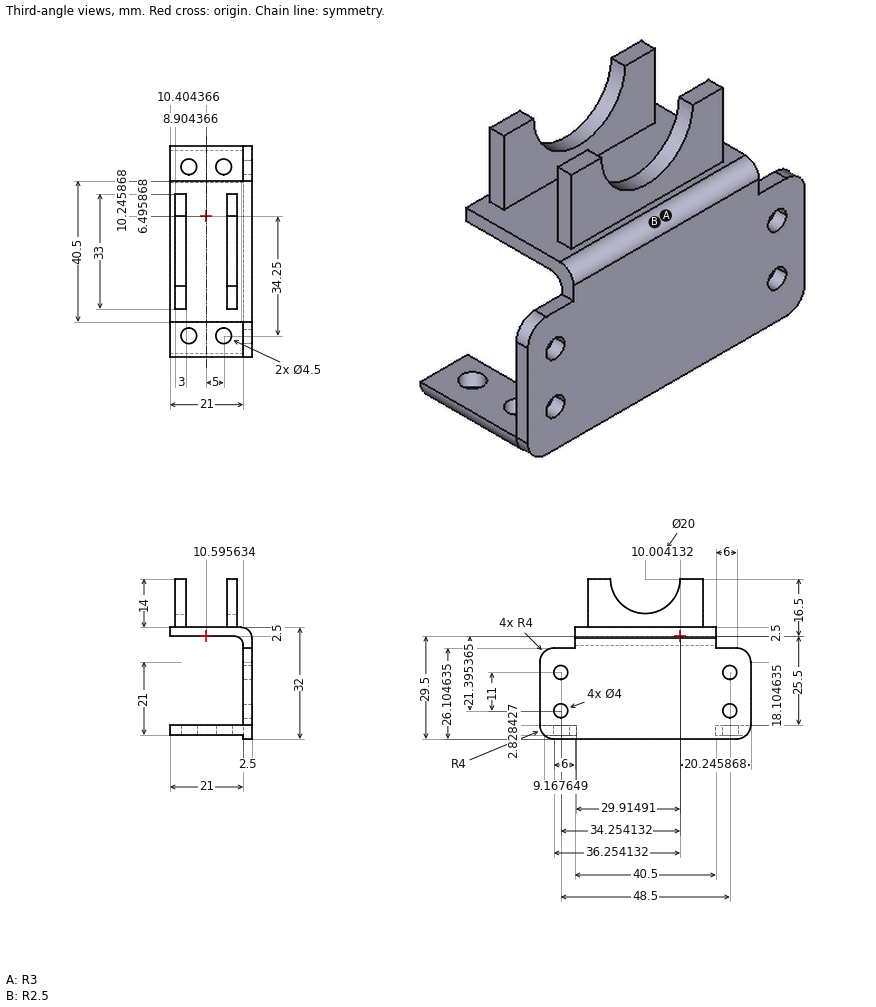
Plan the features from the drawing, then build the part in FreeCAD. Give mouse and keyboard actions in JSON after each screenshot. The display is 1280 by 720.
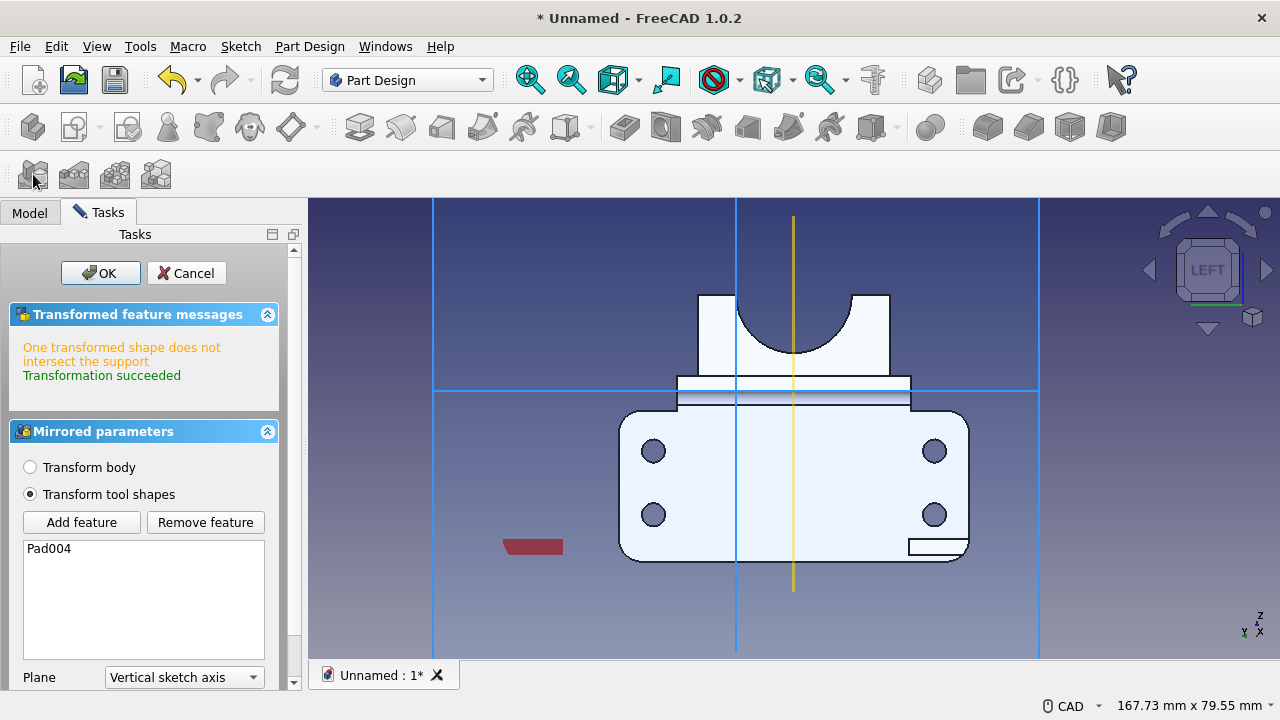
{"action": "left_click", "coordinate": [185, 678]}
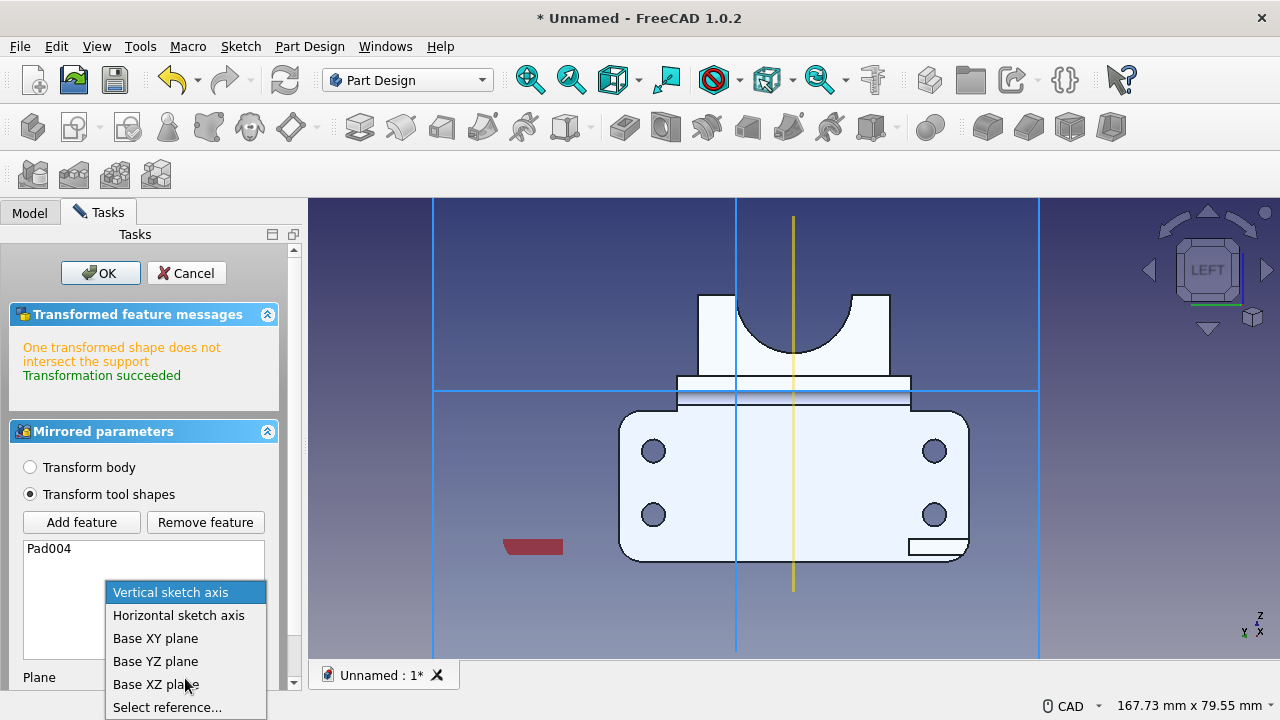
{"action": "left_click", "coordinate": [184, 708]}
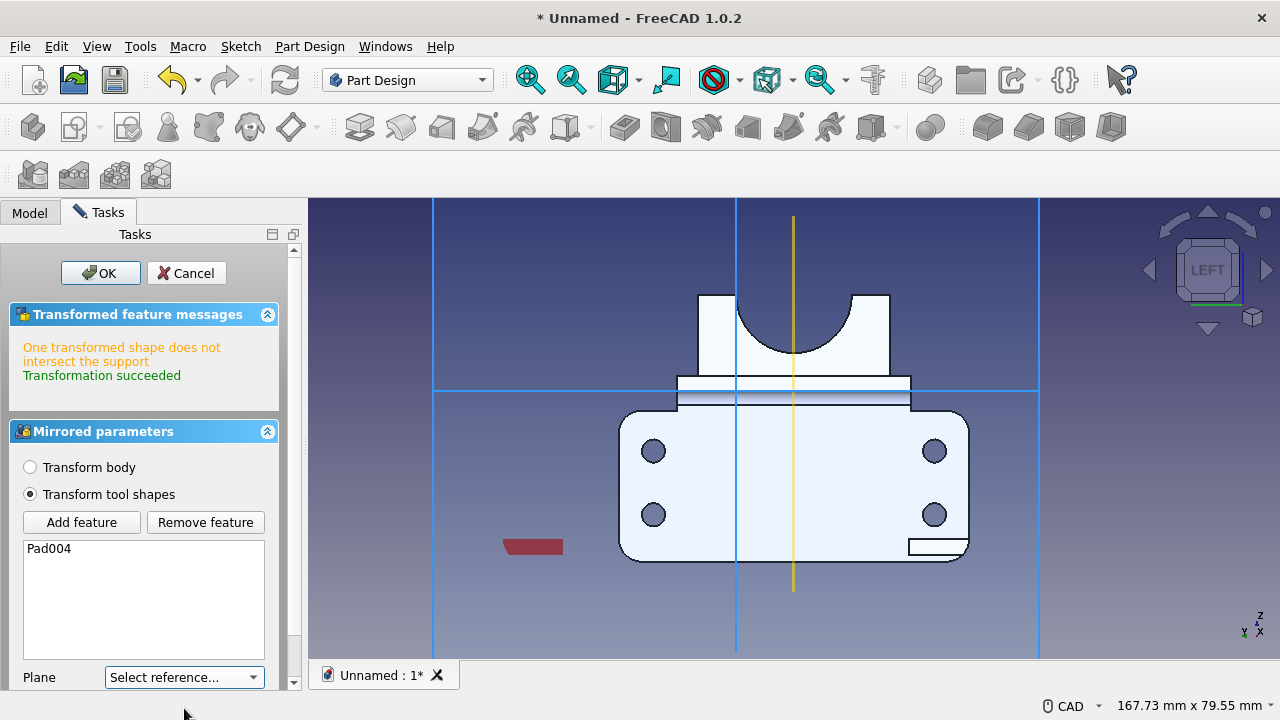
{"action": "left_click", "coordinate": [30, 212]}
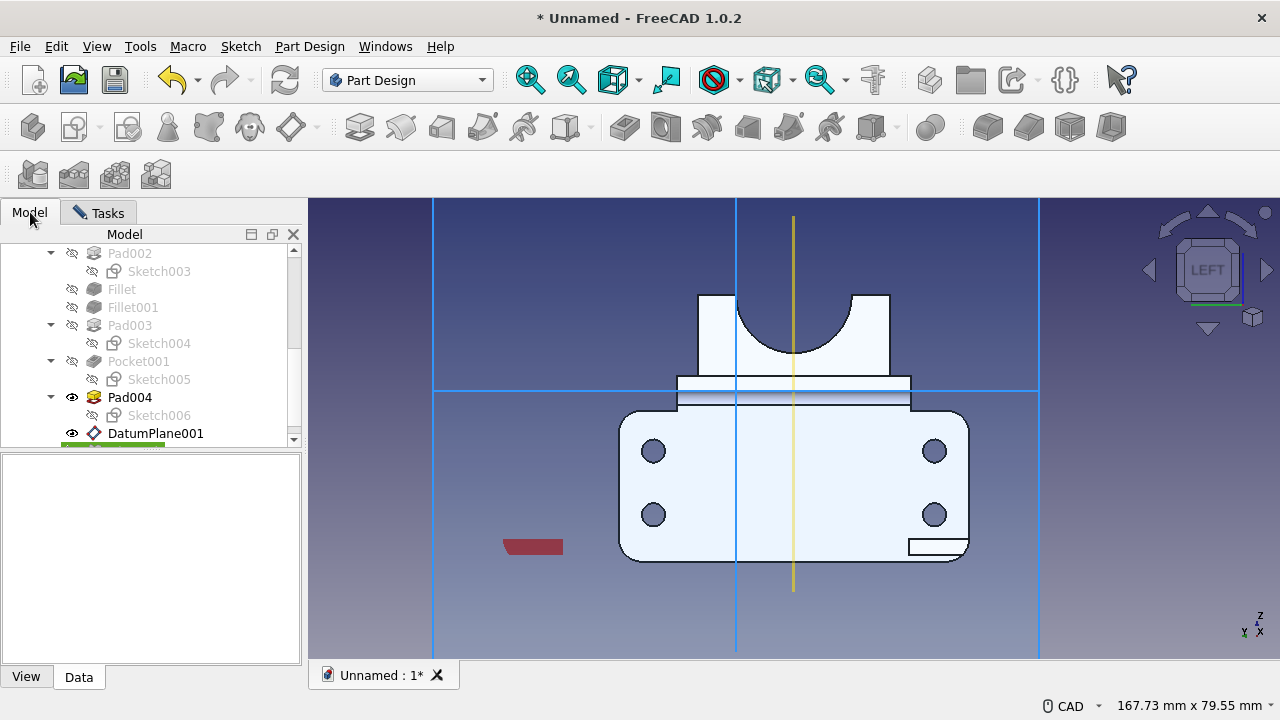
{"action": "left_click", "coordinate": [117, 433]}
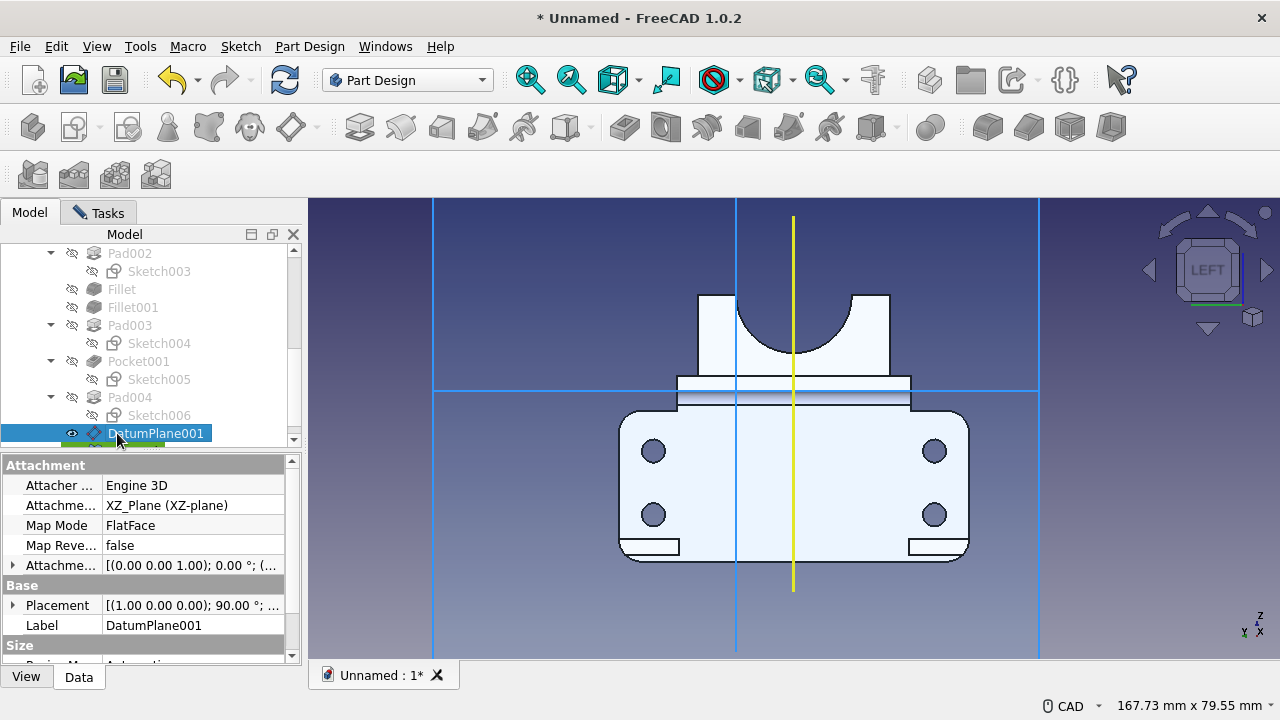
{"action": "left_click", "coordinate": [98, 212]}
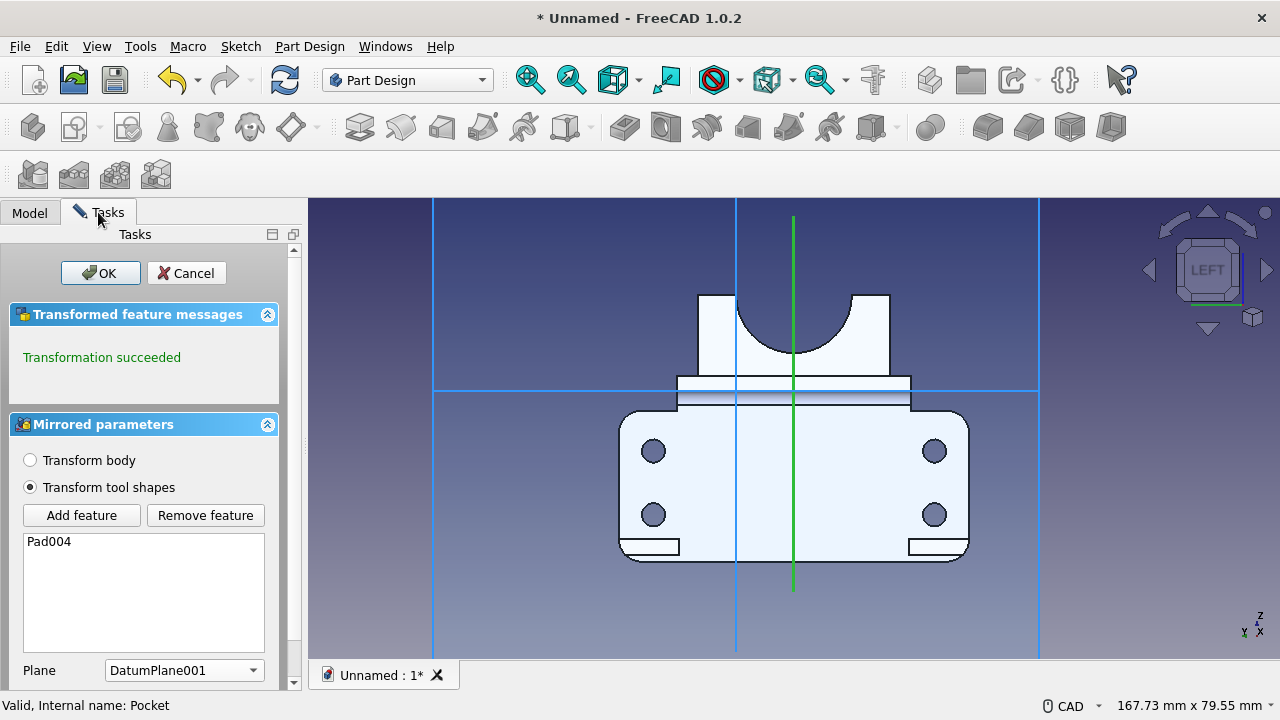
{"action": "left_click", "coordinate": [101, 273]}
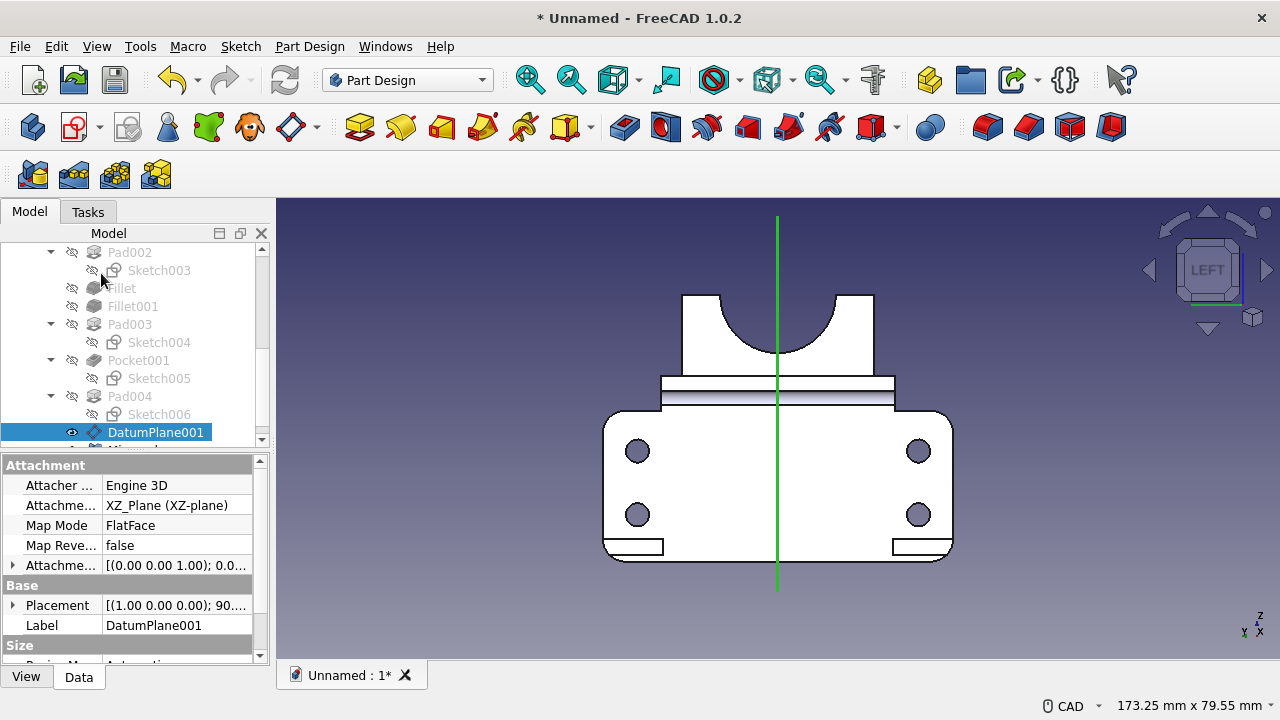
{"action": "left_click", "coordinate": [117, 432]}
{"action": "key", "text": "space"}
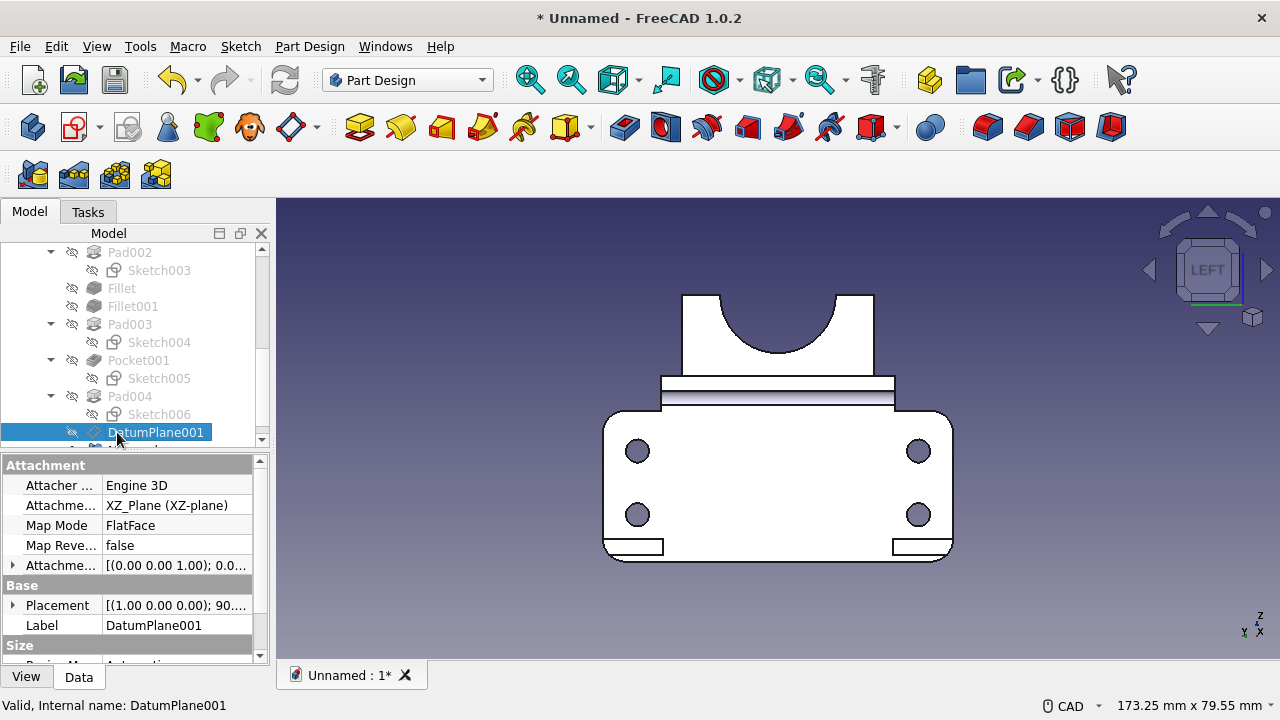
{"action": "key", "text": "5"}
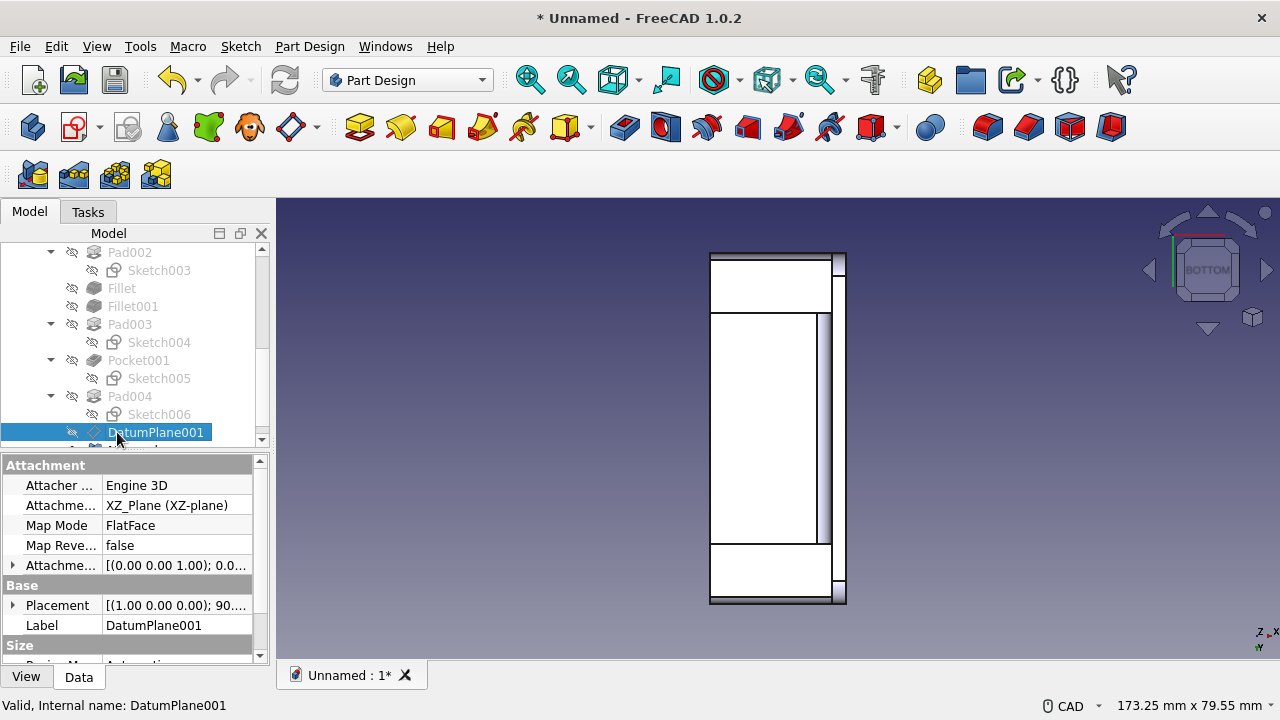
{"action": "left_click", "coordinate": [788, 569]}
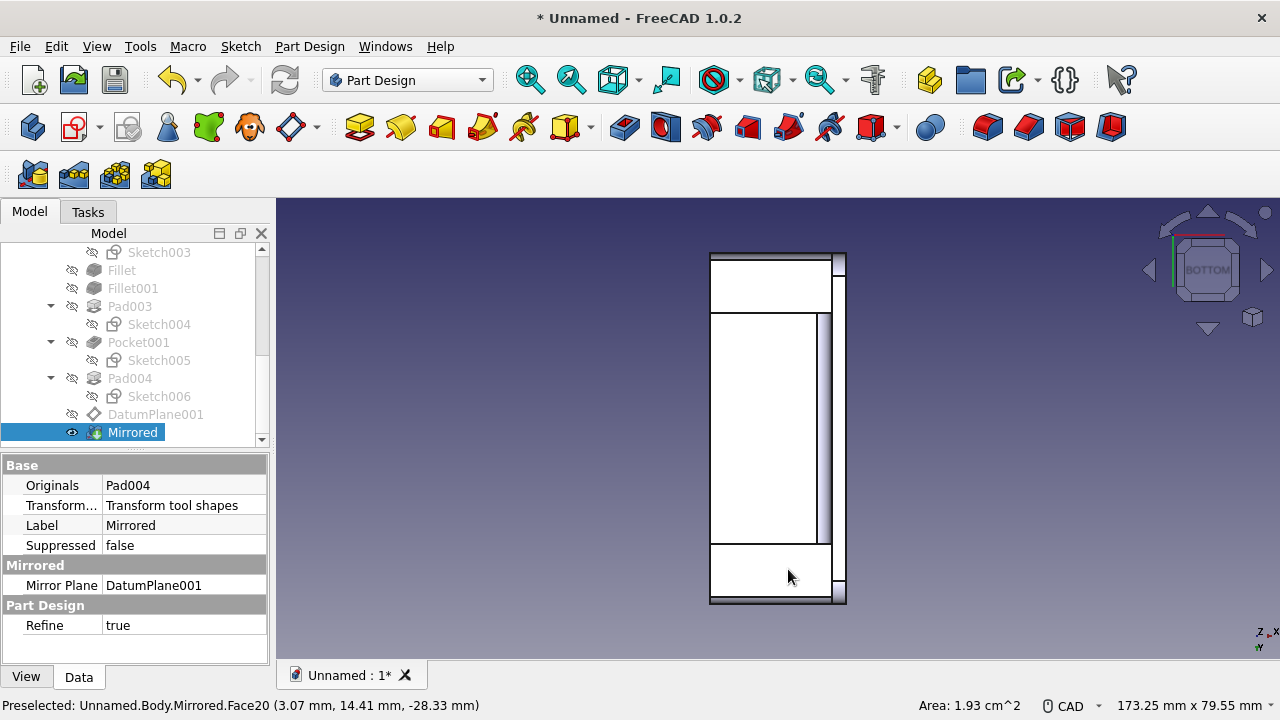
{"action": "left_click", "coordinate": [74, 128]}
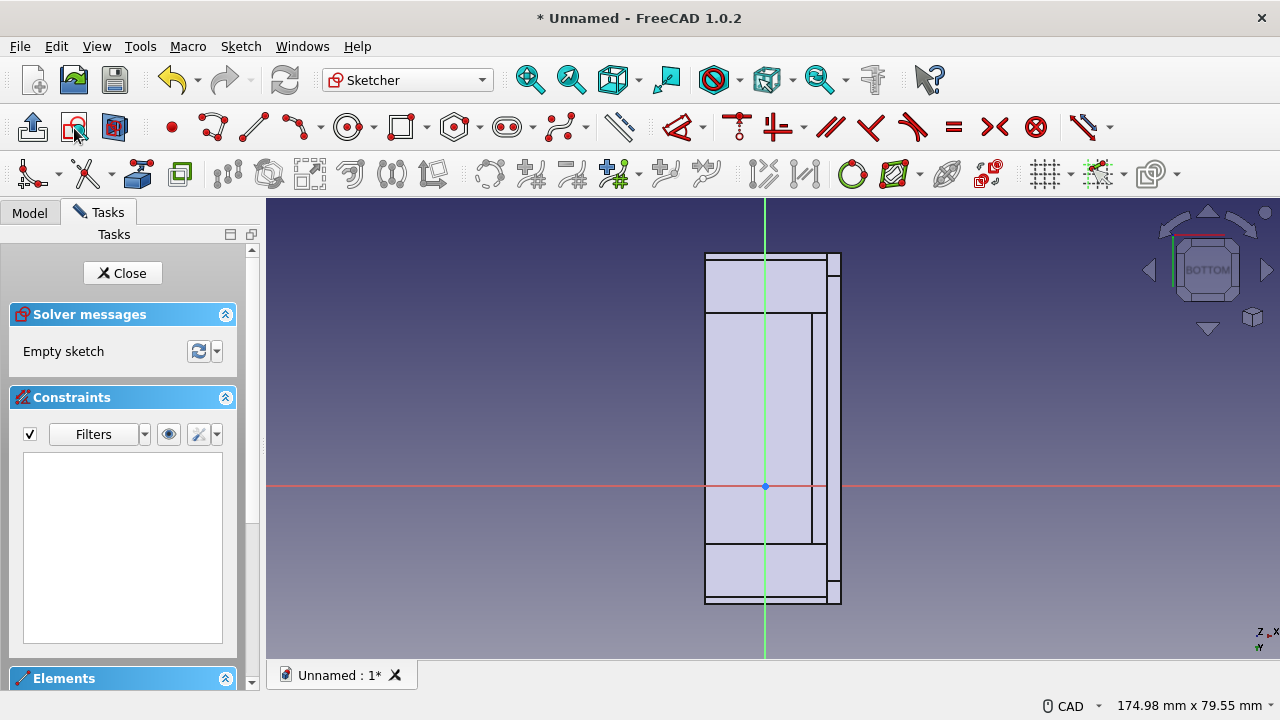
{"action": "scroll", "coordinate": [775, 266], "scroll_direction": "up", "scroll_amount": 10}